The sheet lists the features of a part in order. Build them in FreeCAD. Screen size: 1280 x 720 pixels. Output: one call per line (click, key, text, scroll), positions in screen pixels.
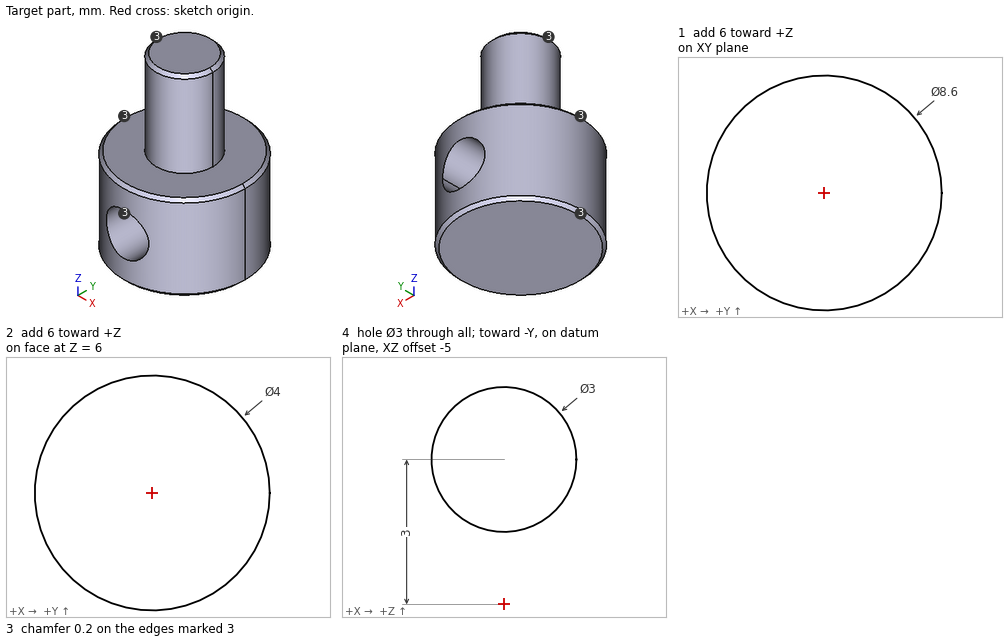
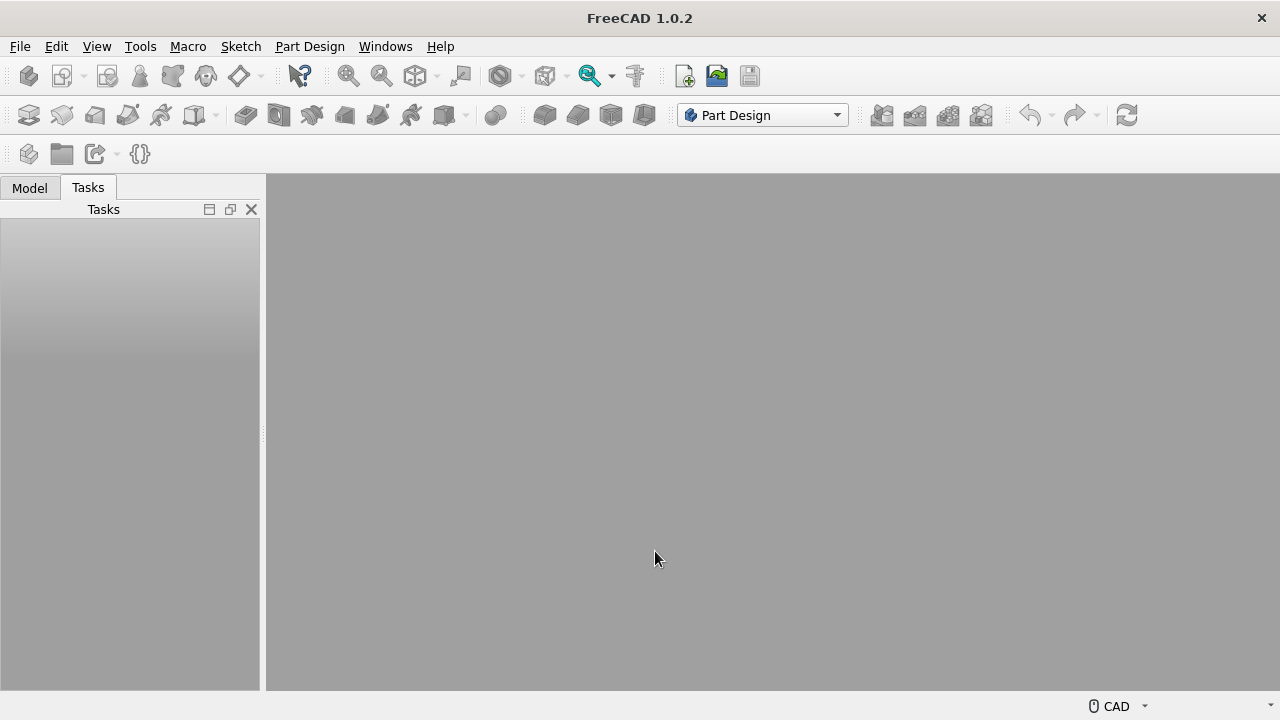
key(ctrl+n)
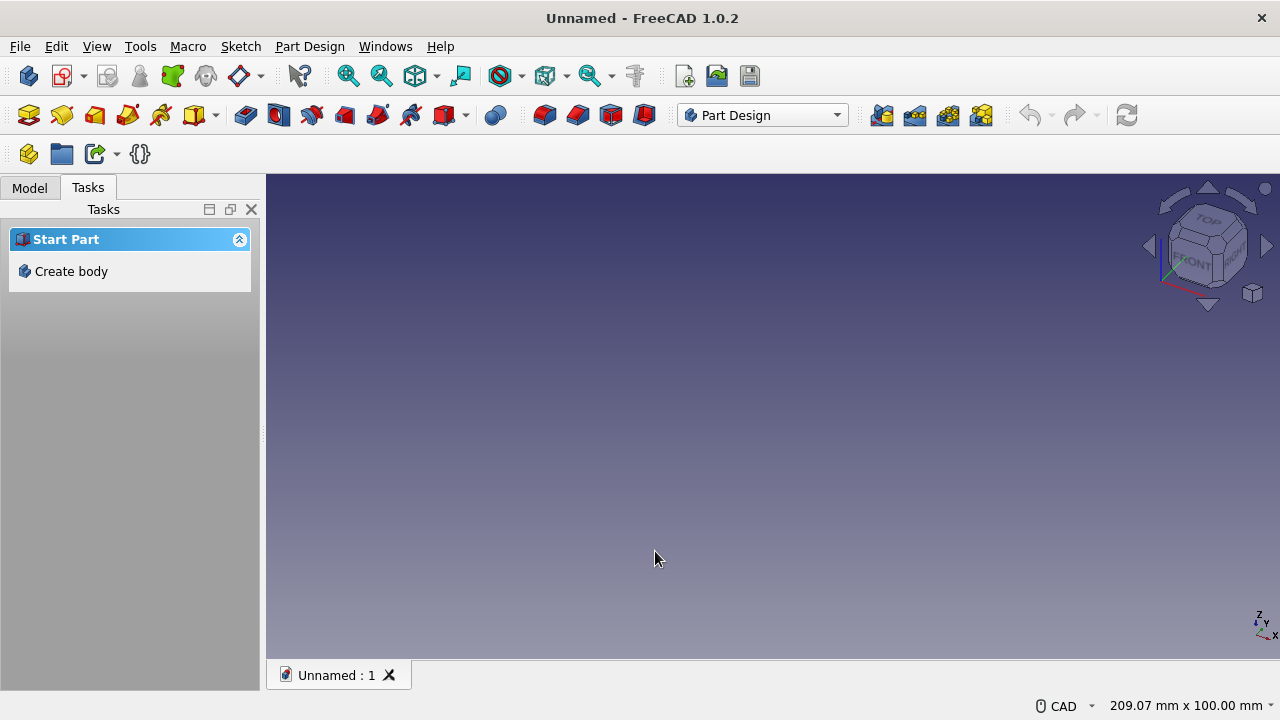
click(62, 76)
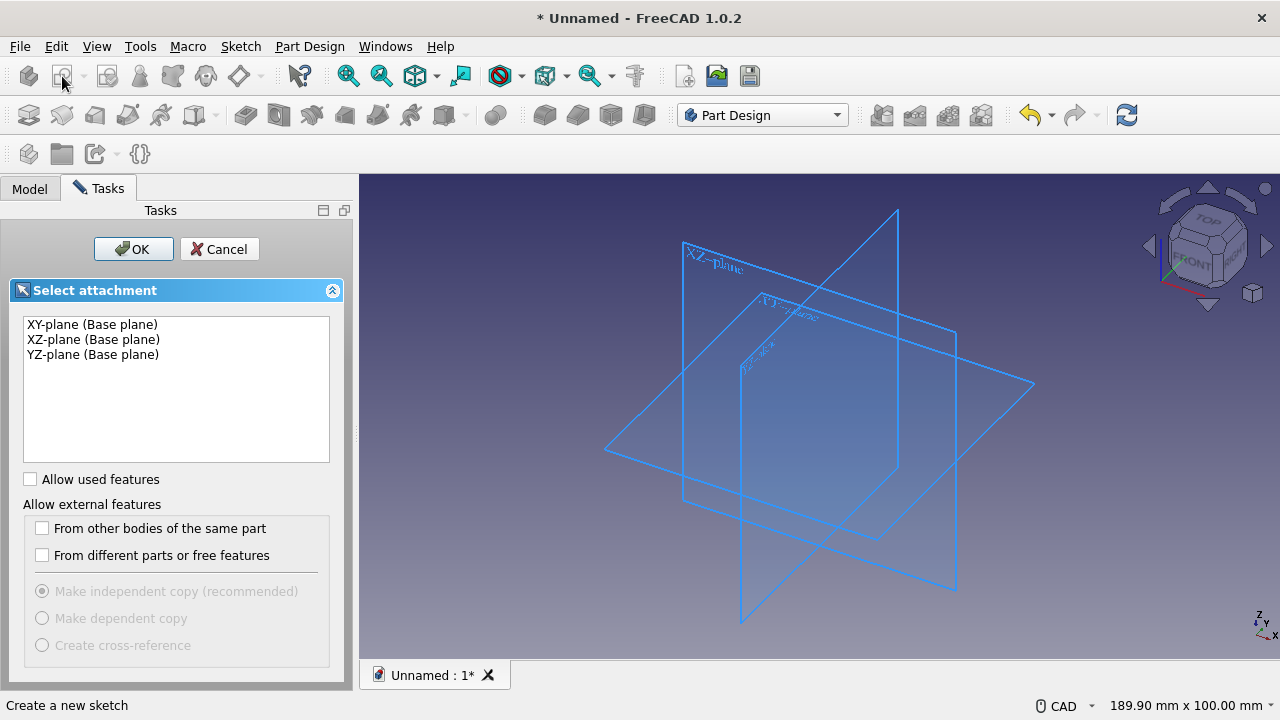
click(84, 324)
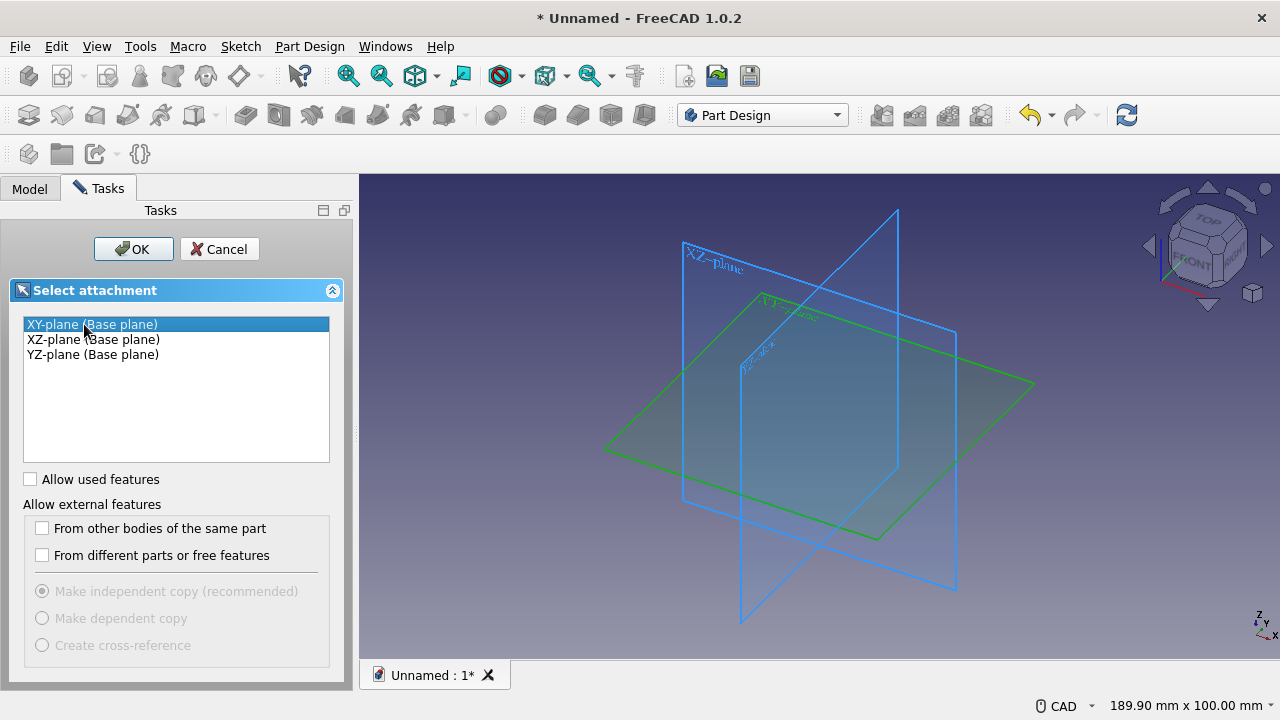
click(134, 249)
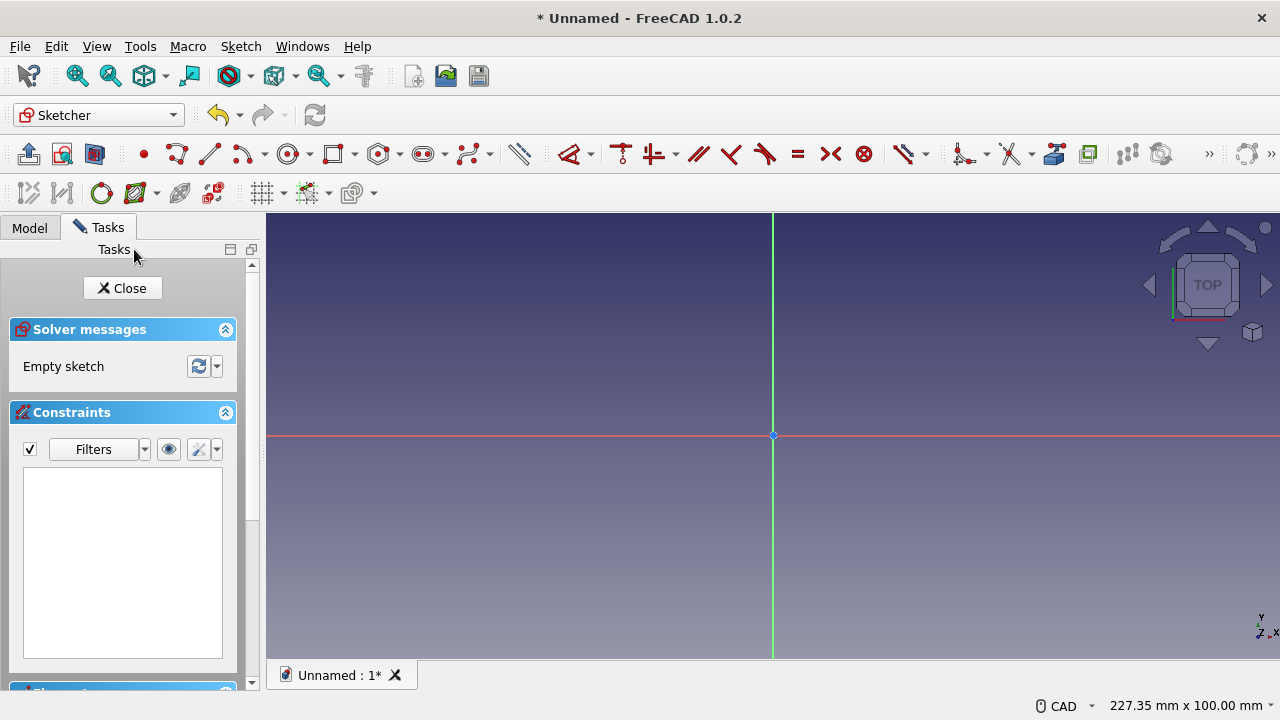
scroll(784, 436, up, 10)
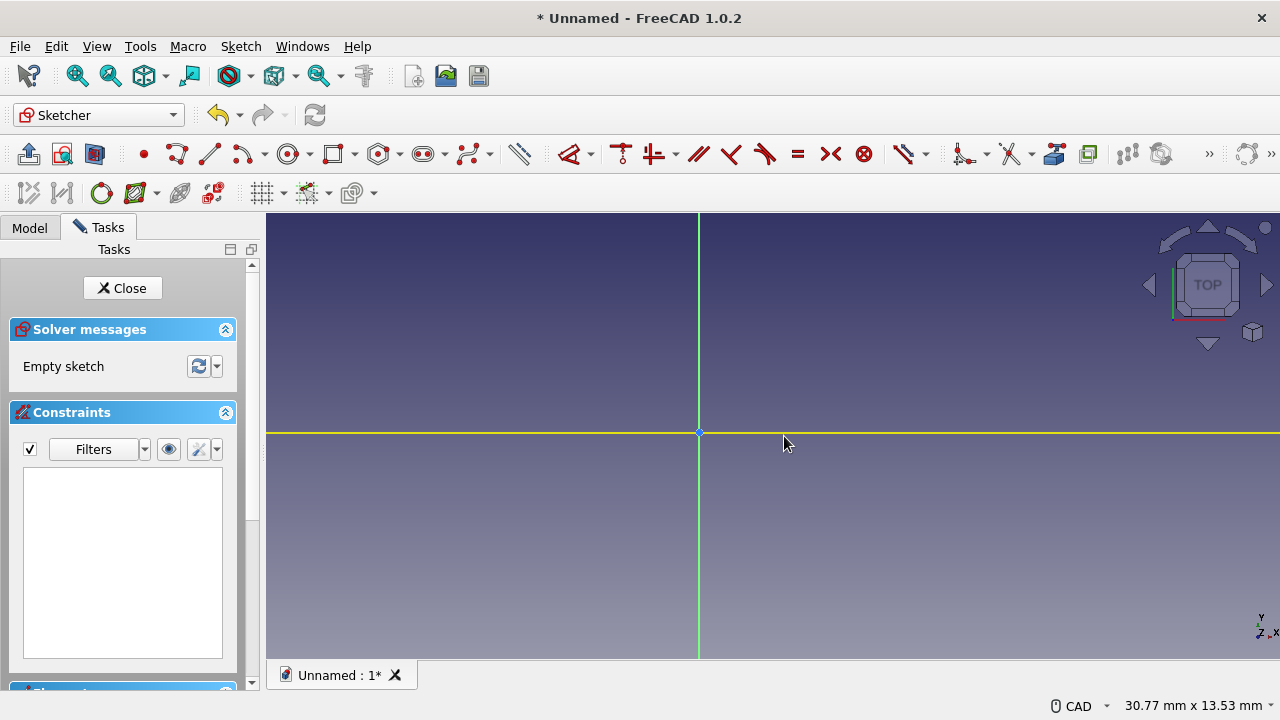
key(g)
key(c)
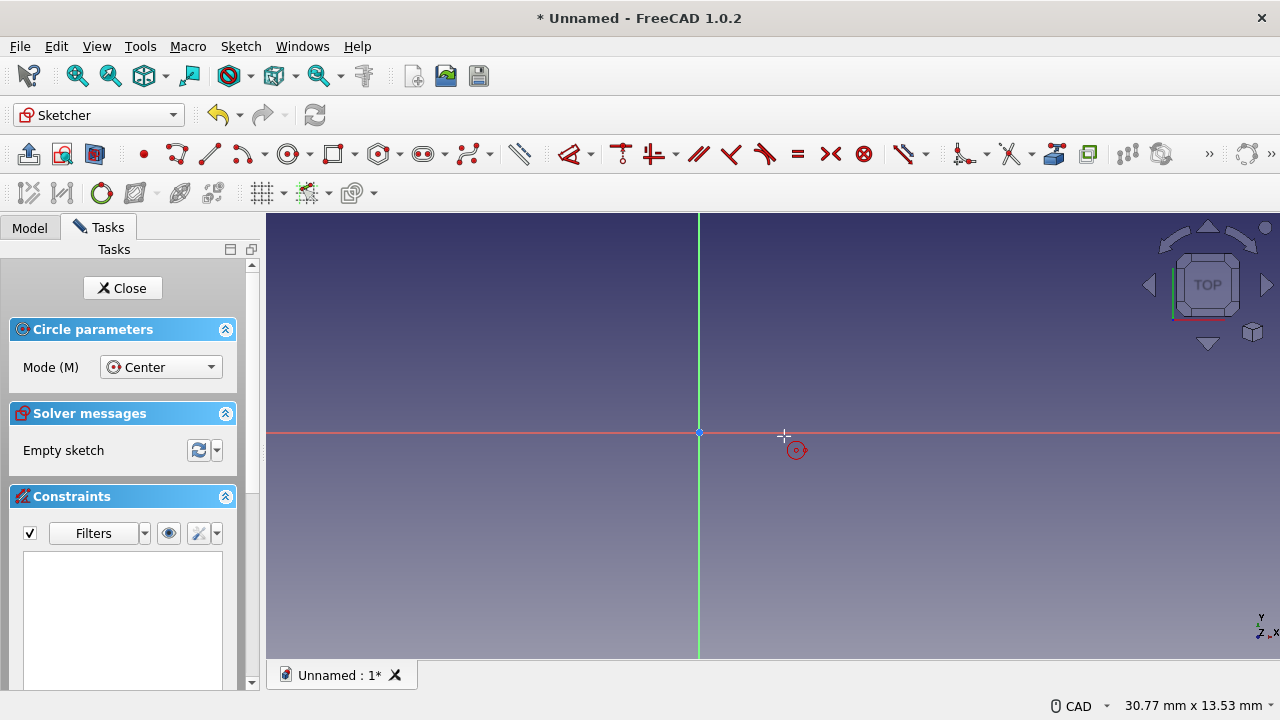
click(699, 433)
move(800, 333)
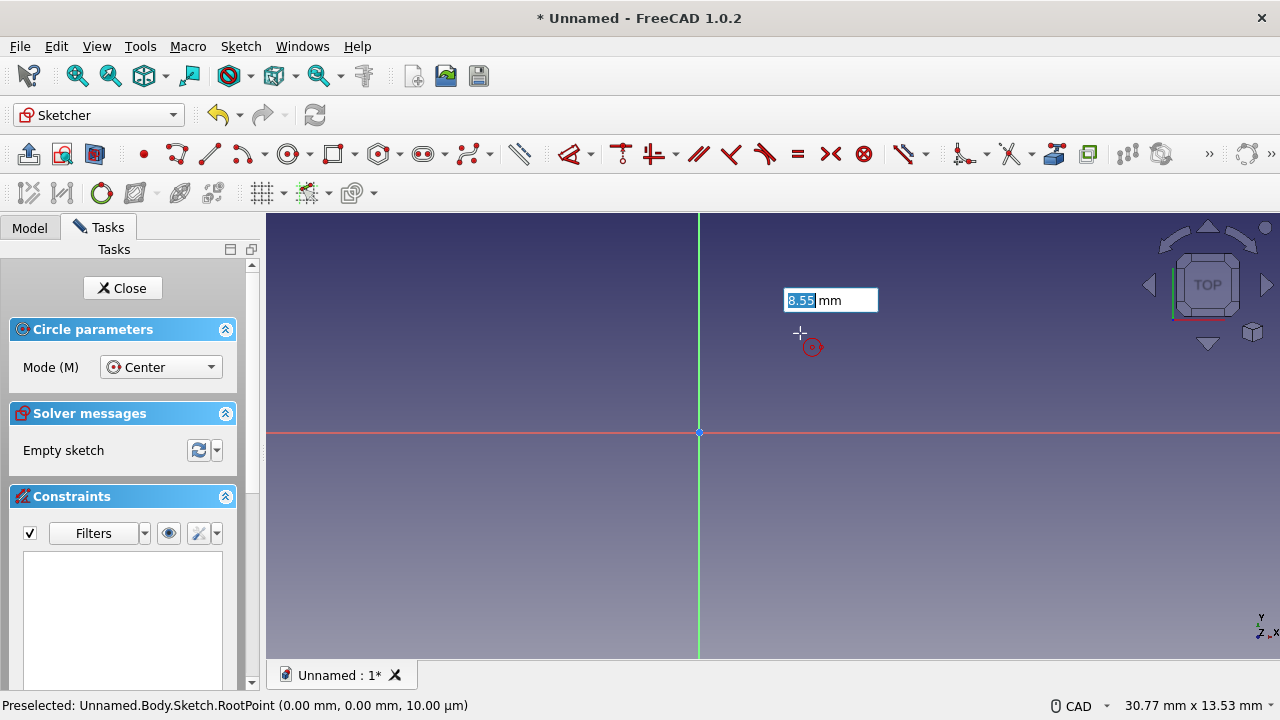
text(8.6)
key(Return)
key(Escape)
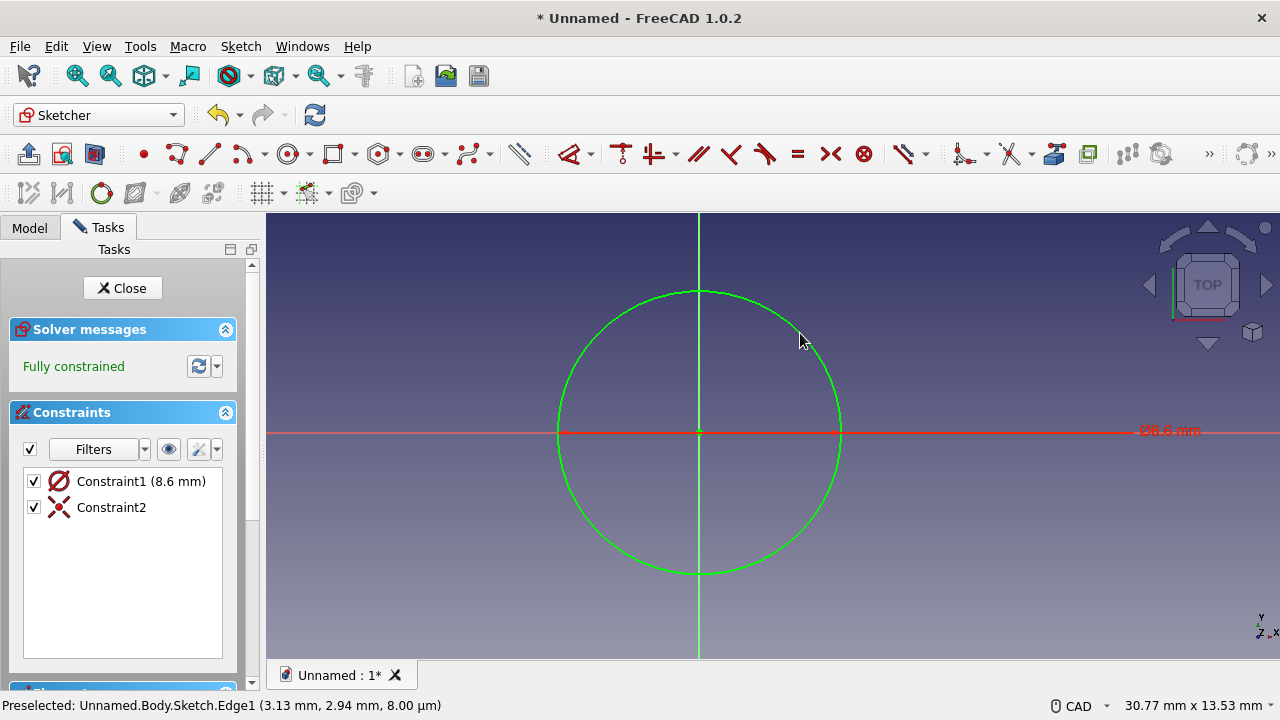
click(123, 288)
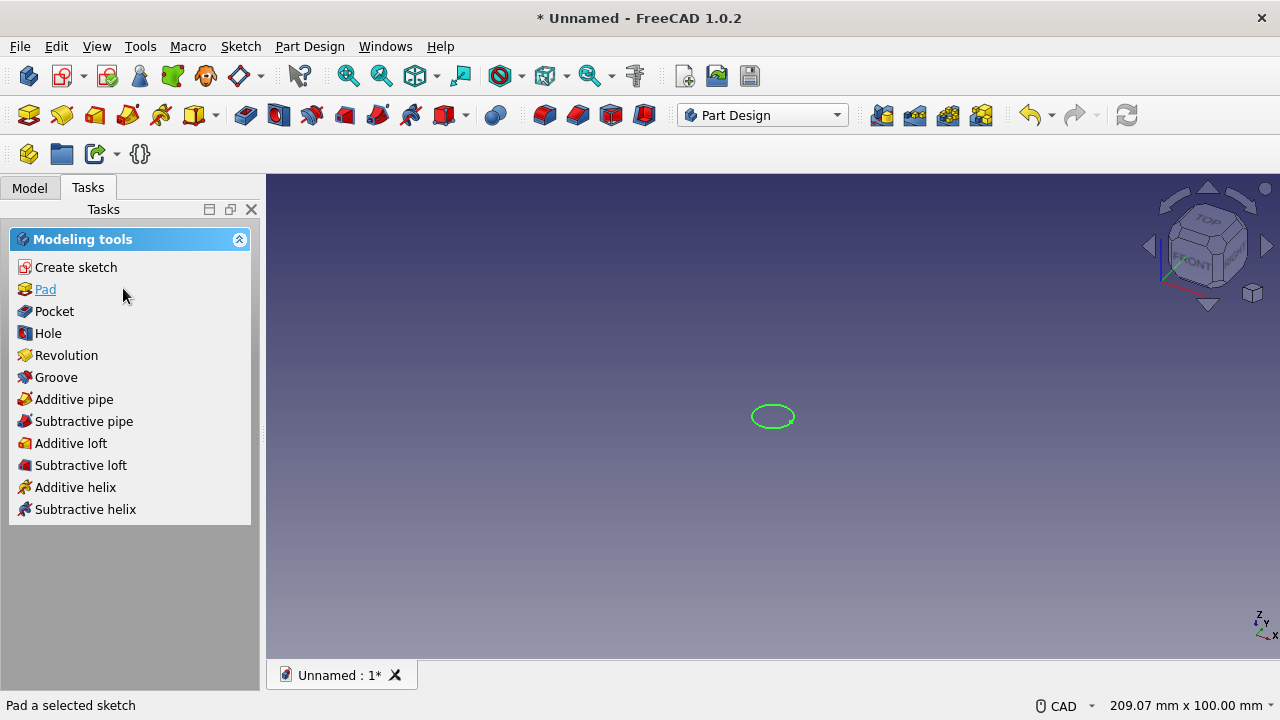
click(29, 116)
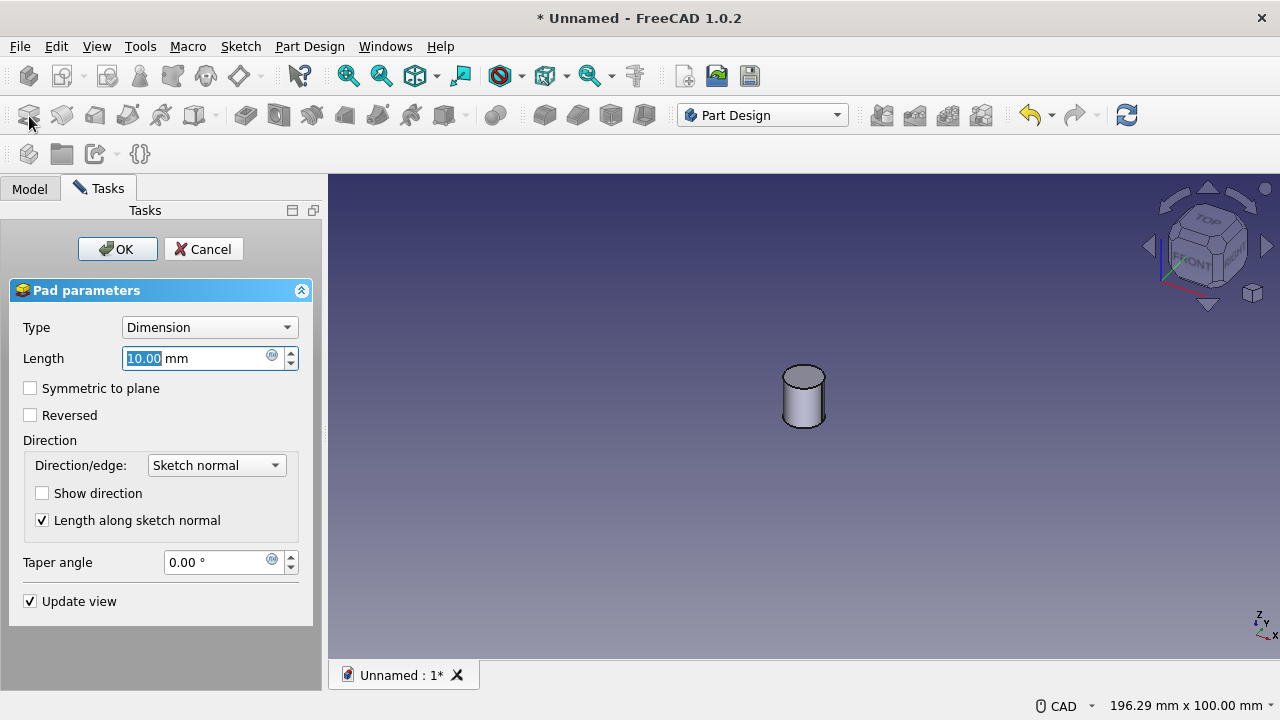
text(6)
key(Tab)